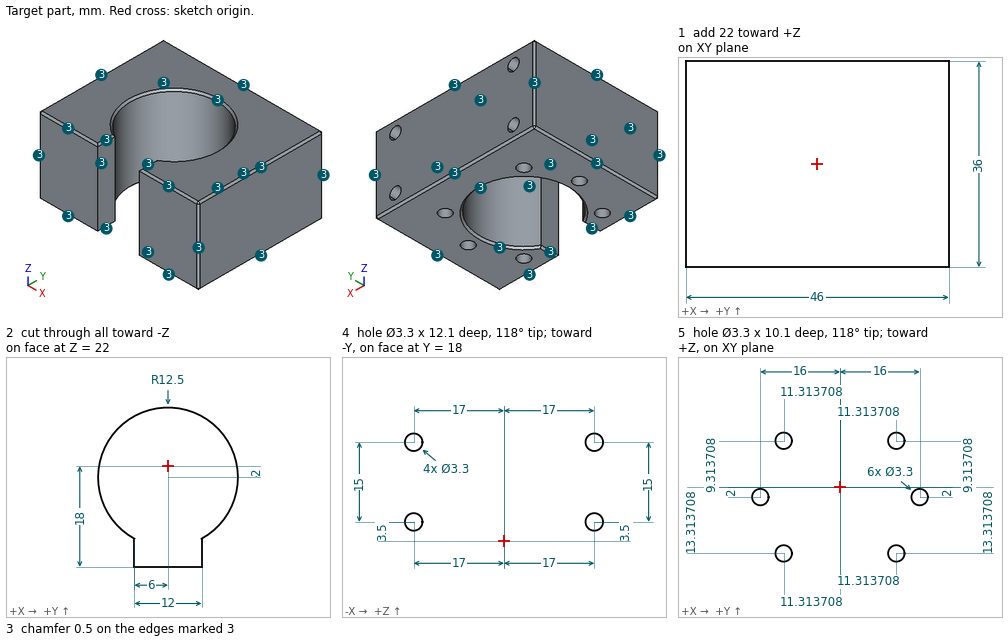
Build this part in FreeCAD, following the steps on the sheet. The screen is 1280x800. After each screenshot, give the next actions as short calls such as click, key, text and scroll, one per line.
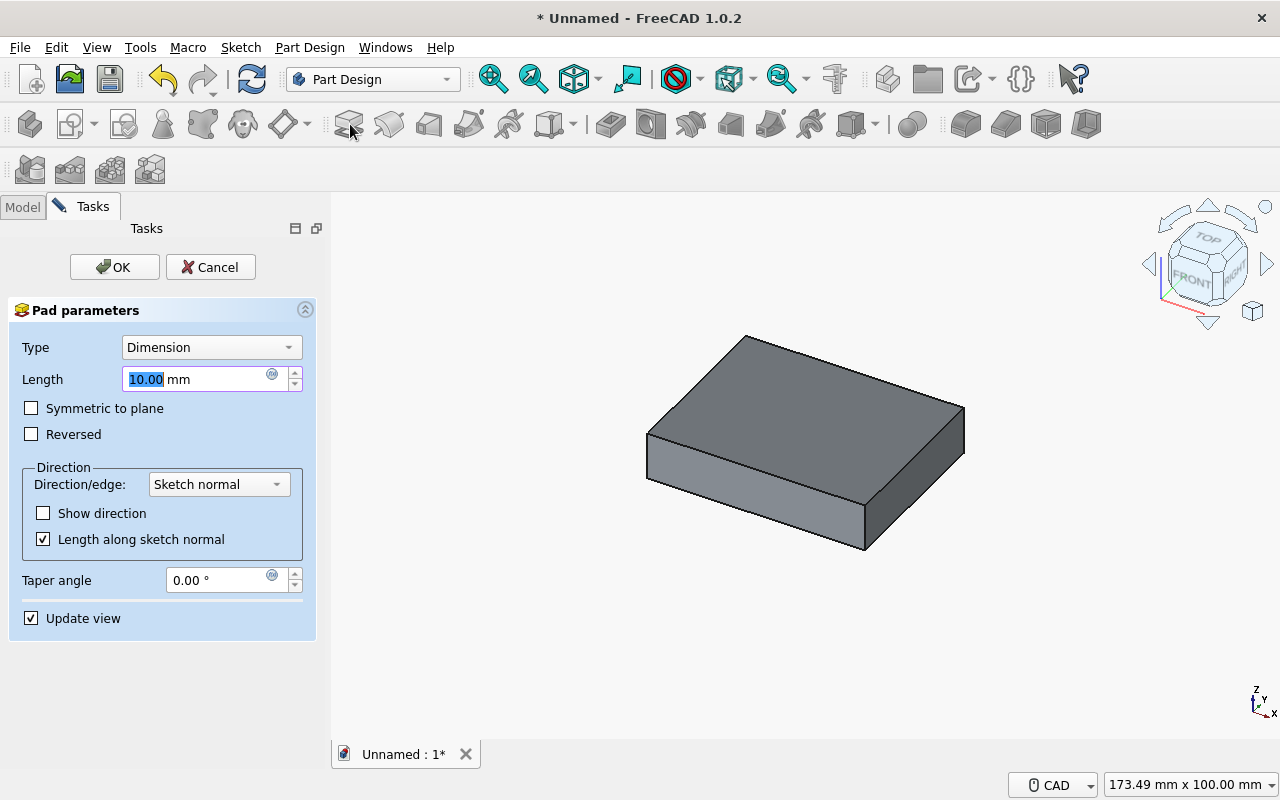
text(22)
key(Tab)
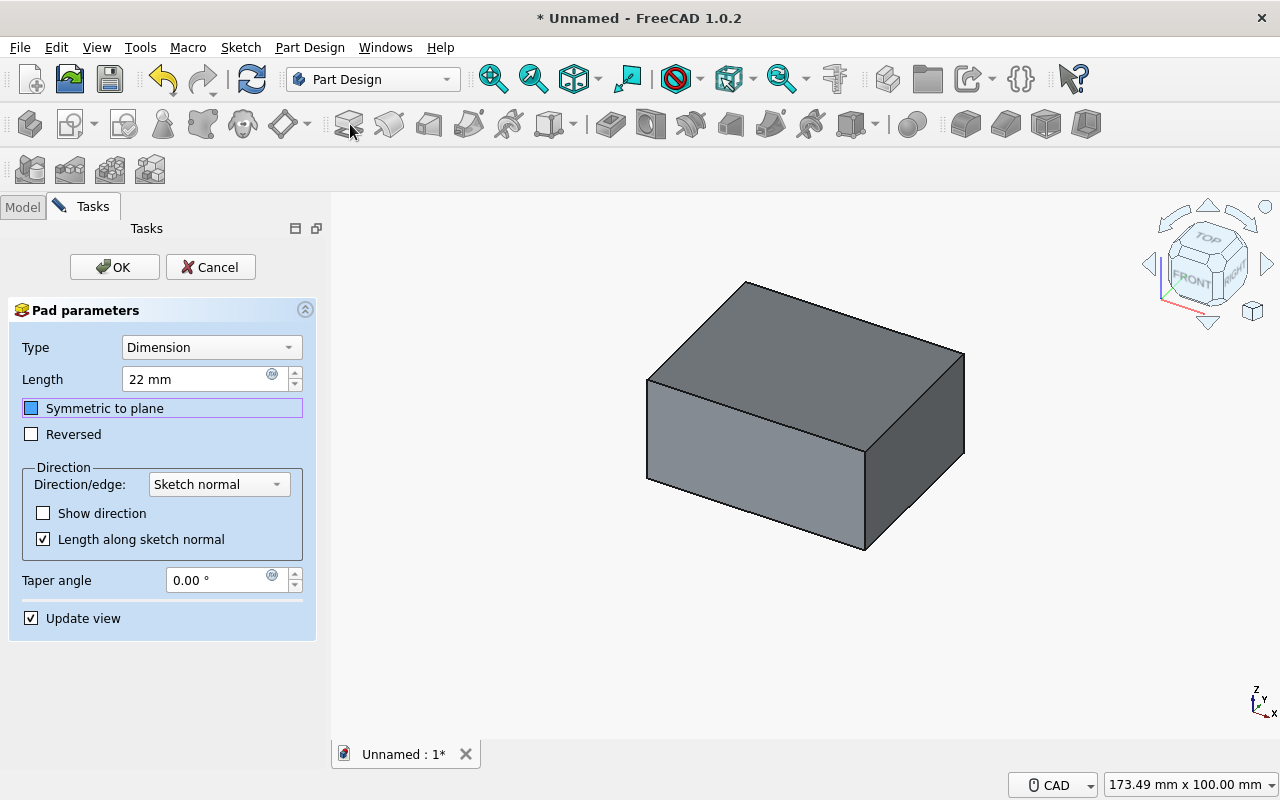
click(115, 267)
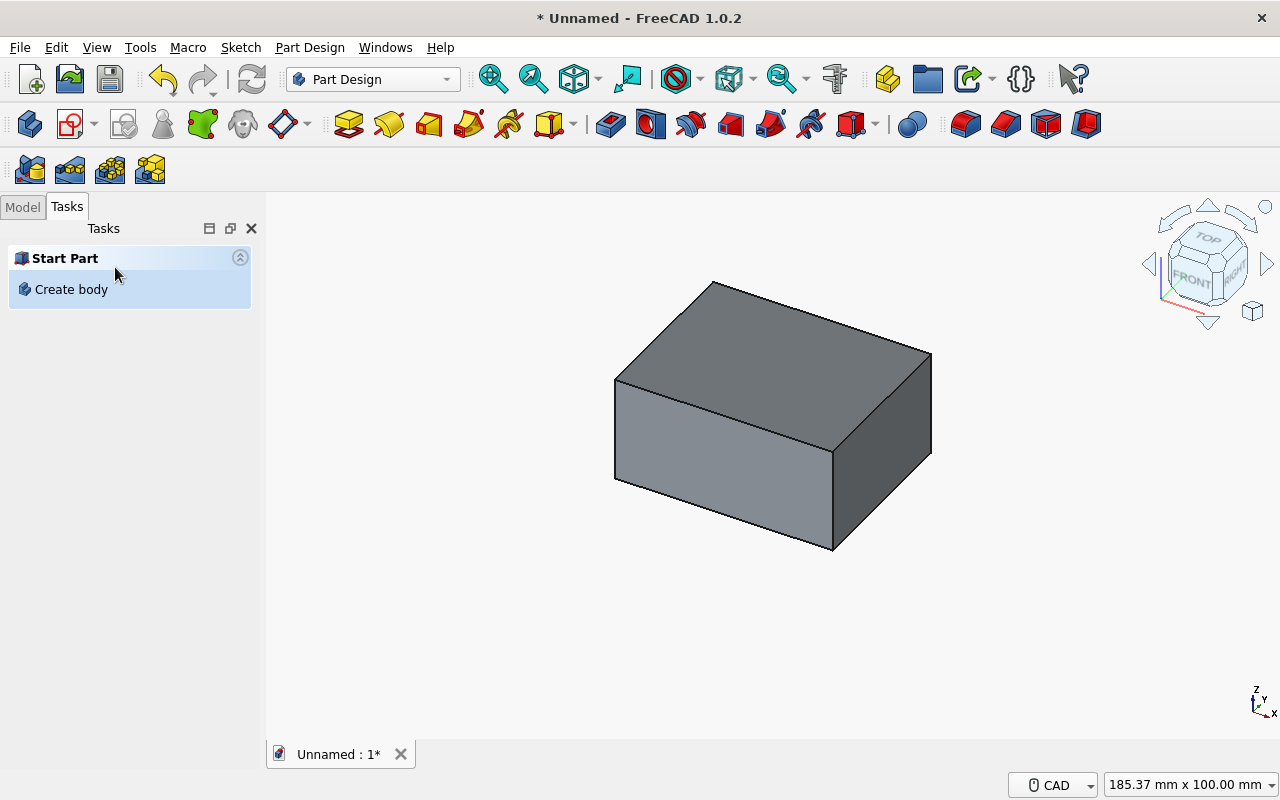
click(773, 366)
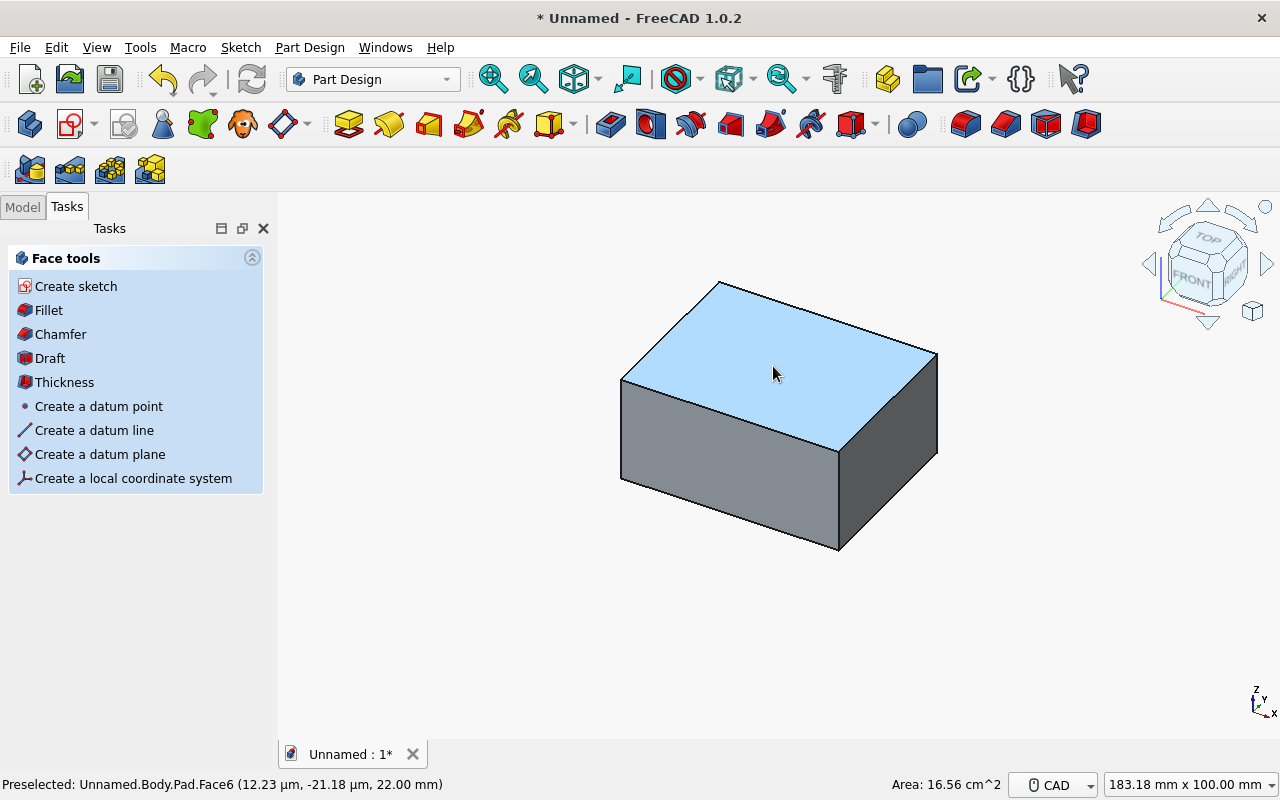
click(70, 124)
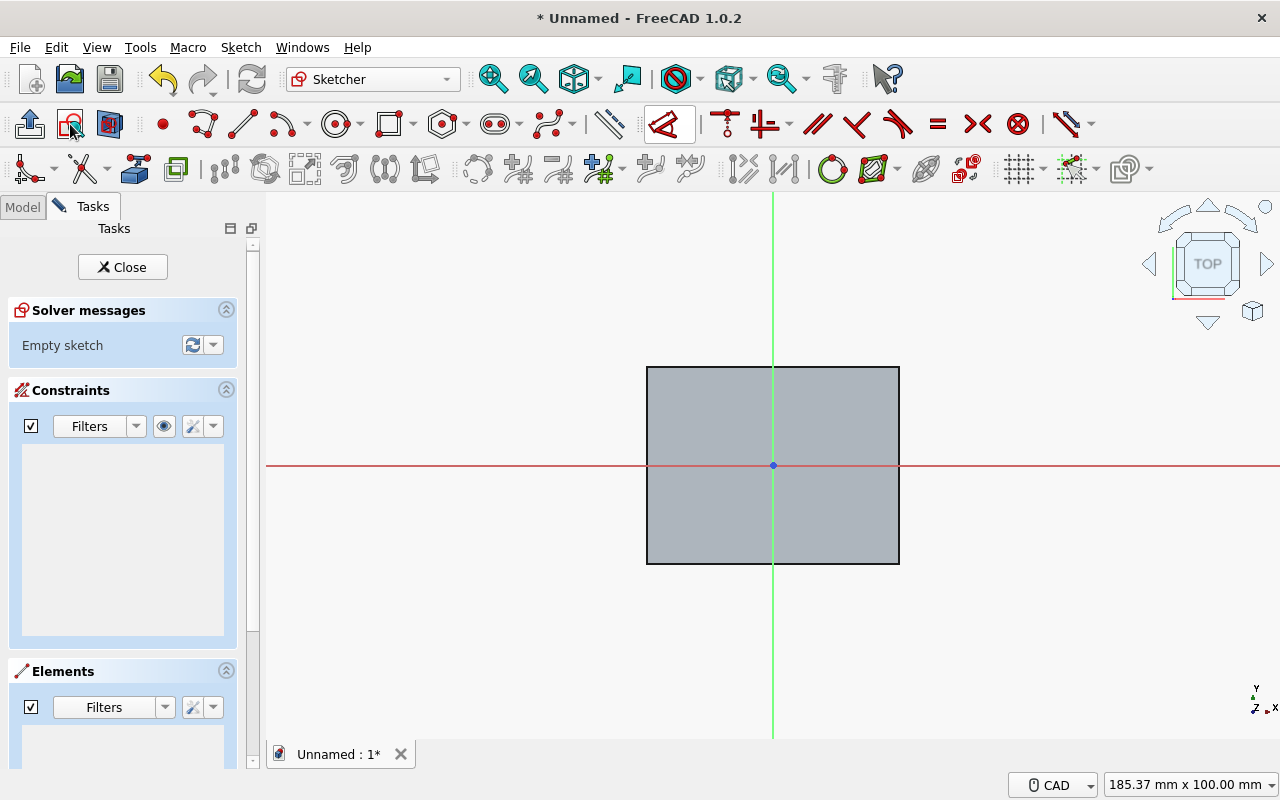
scroll(829, 503, up, 4)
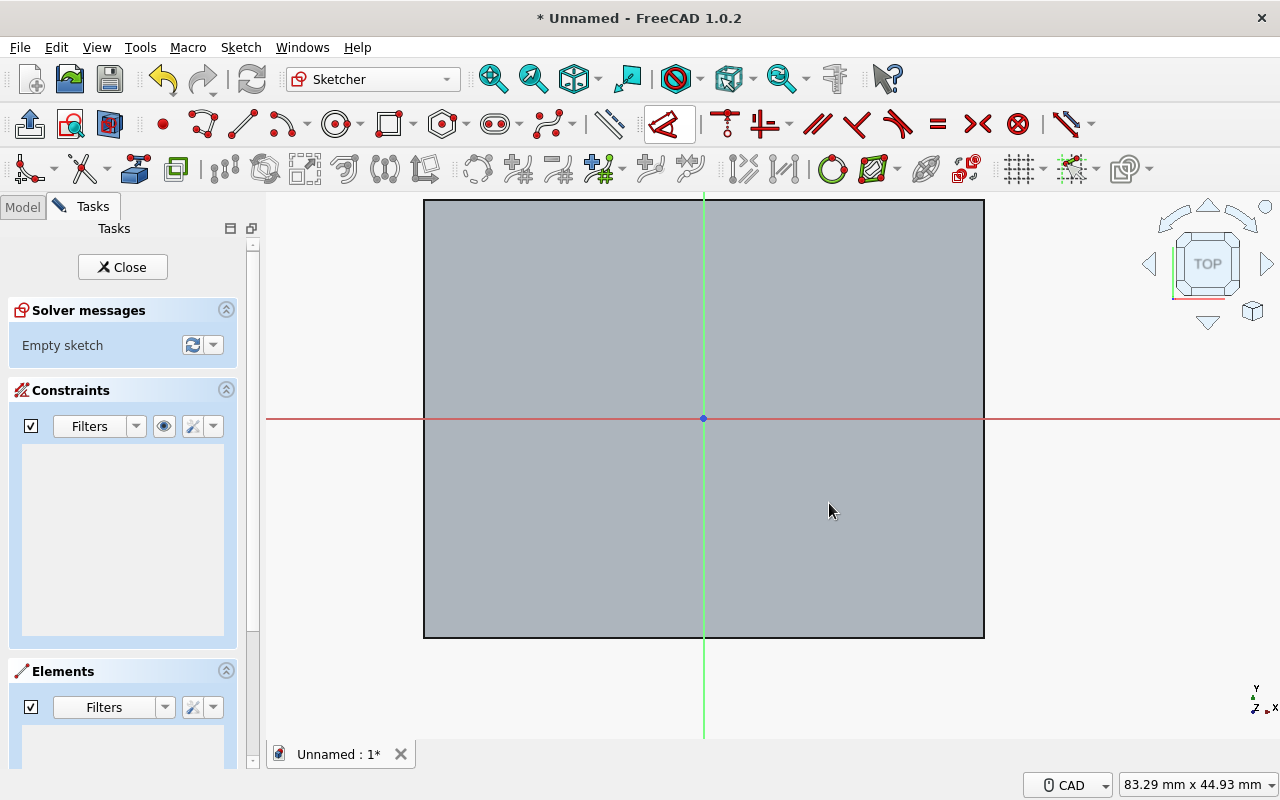
key(g)
key(m)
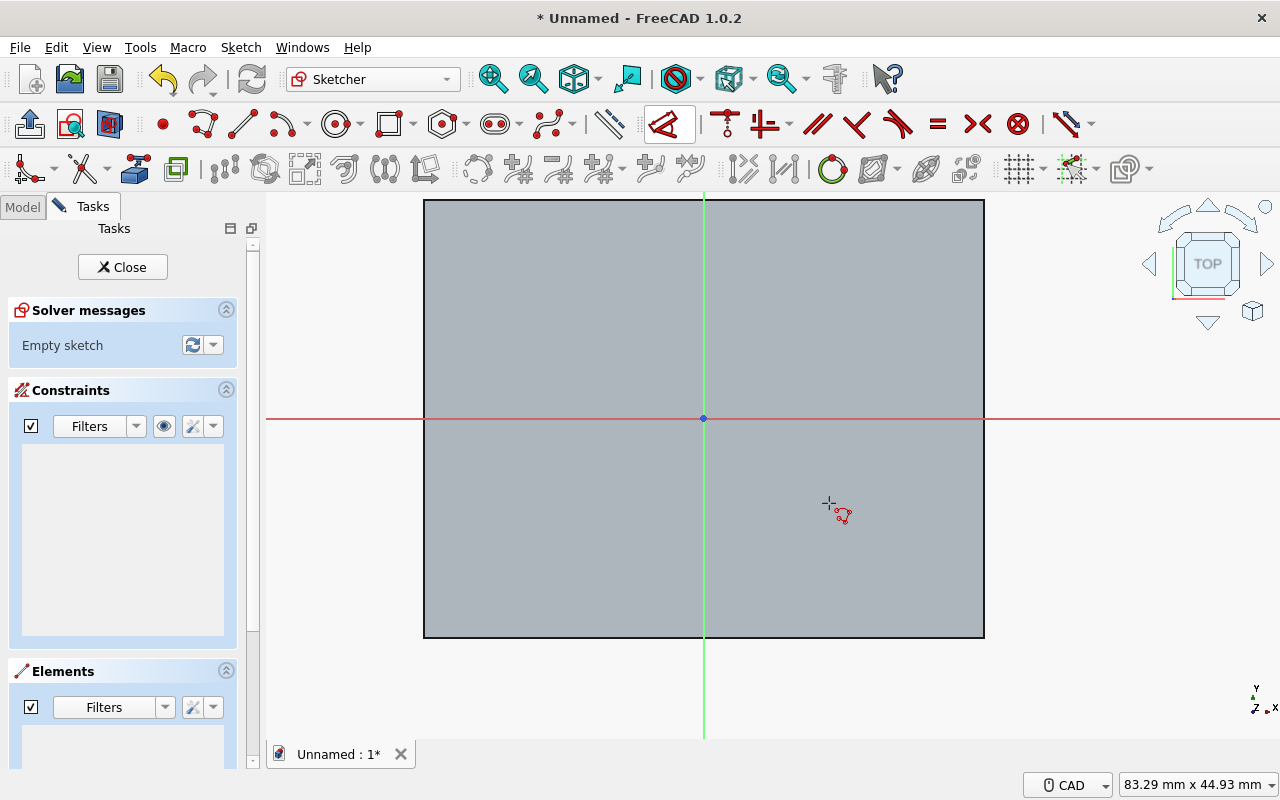
click(631, 577)
click(631, 638)
click(777, 638)
click(777, 577)
right_click(777, 577)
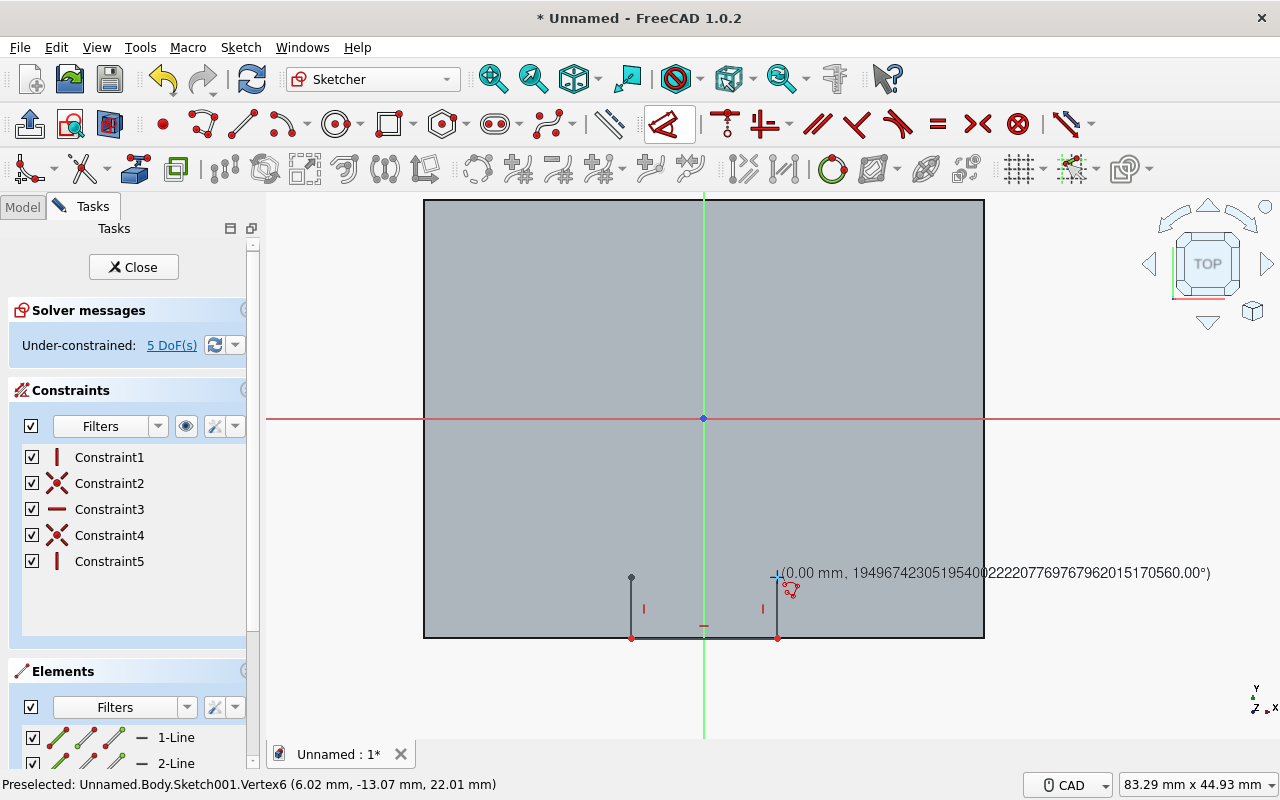
key(g)
key(3)
key(a)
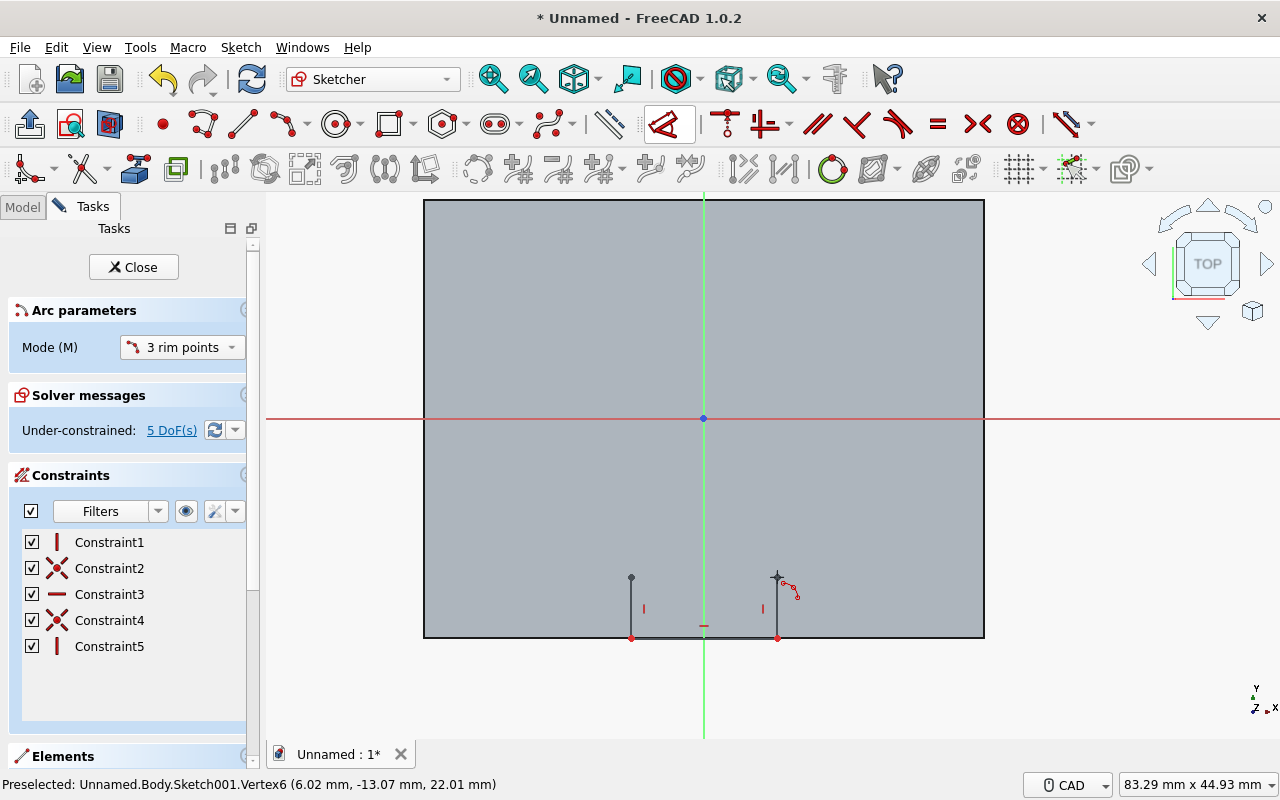
click(777, 578)
click(631, 578)
click(780, 312)
key(Escape)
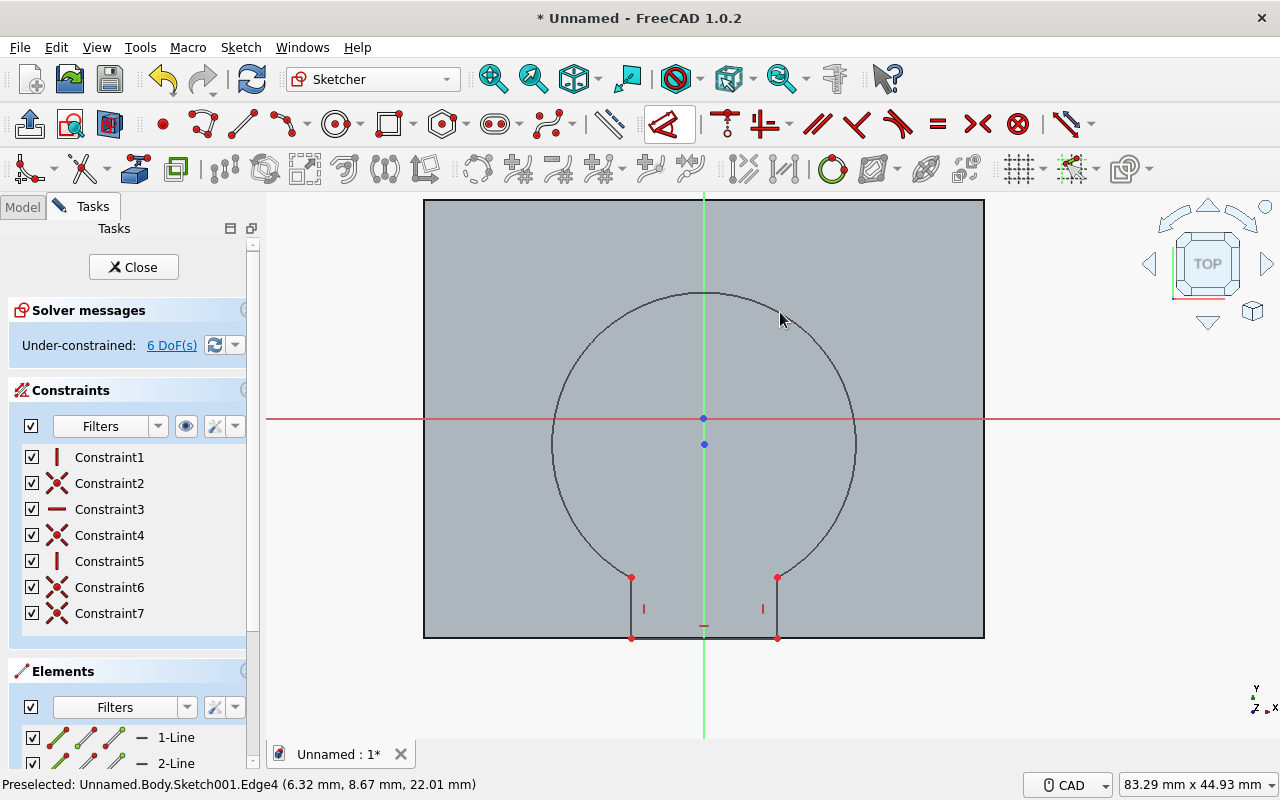
click(704, 445)